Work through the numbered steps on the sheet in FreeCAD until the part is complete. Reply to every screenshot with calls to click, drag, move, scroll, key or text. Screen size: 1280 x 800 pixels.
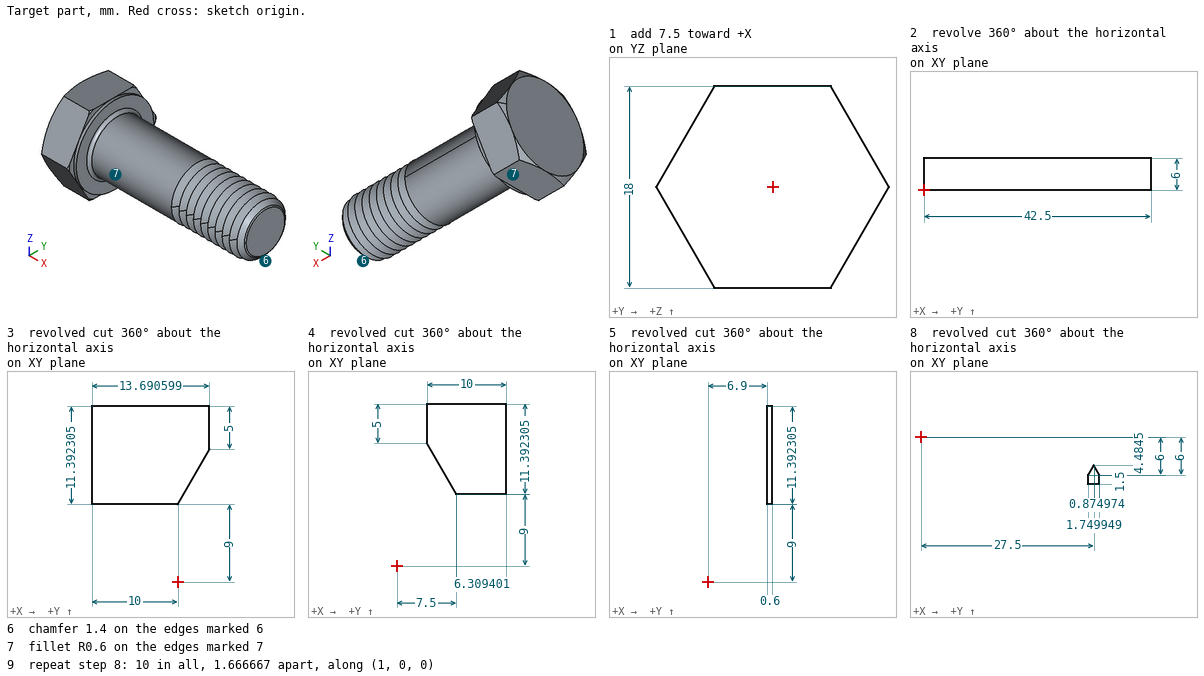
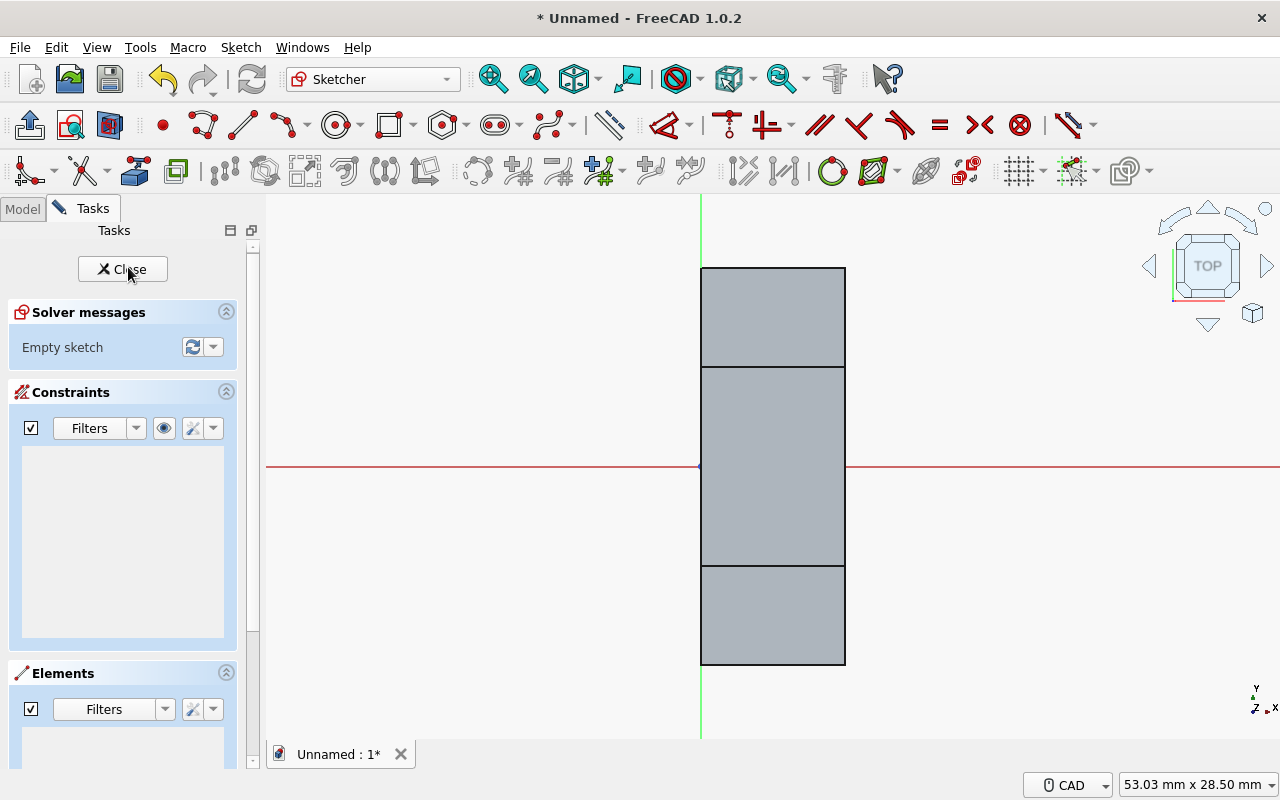
key(q)
key(s)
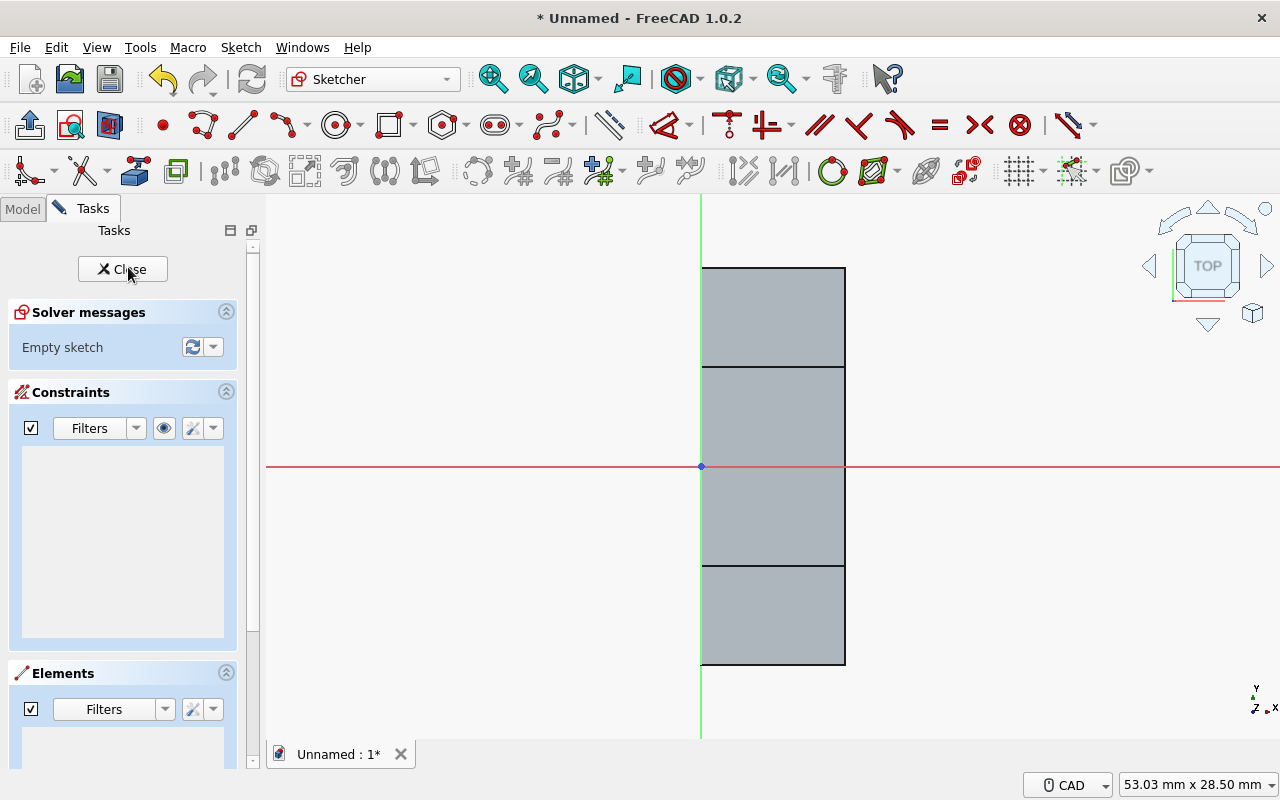
scroll(294, 536, down, 3)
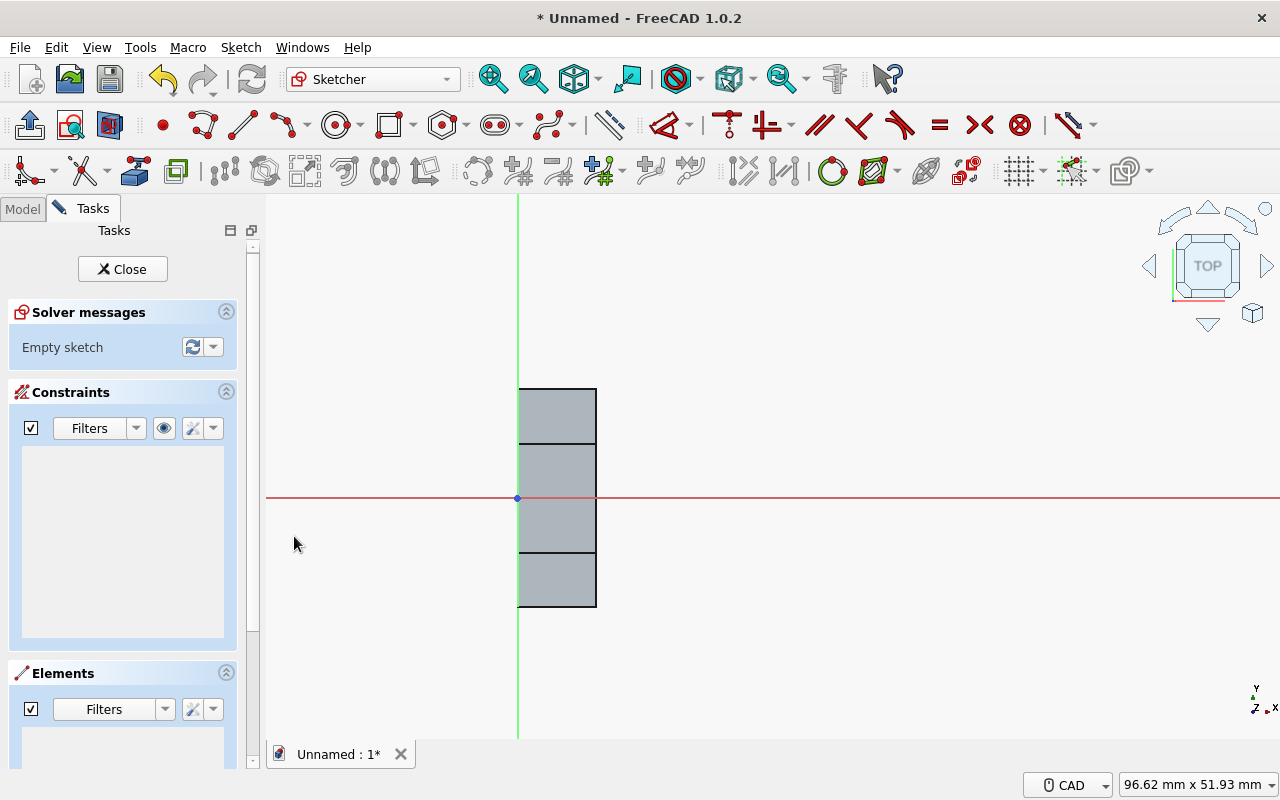
key(g)
key(r)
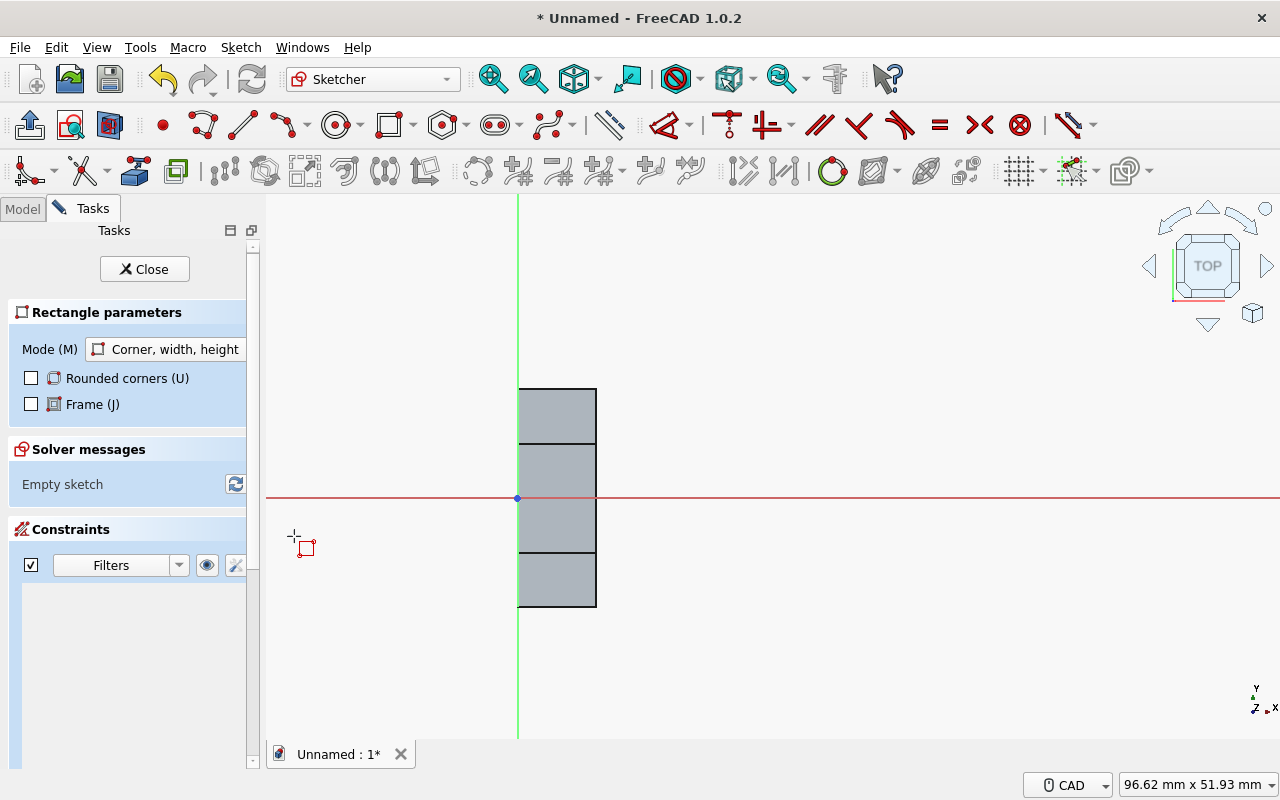
click(518, 498)
click(964, 435)
key(Escape)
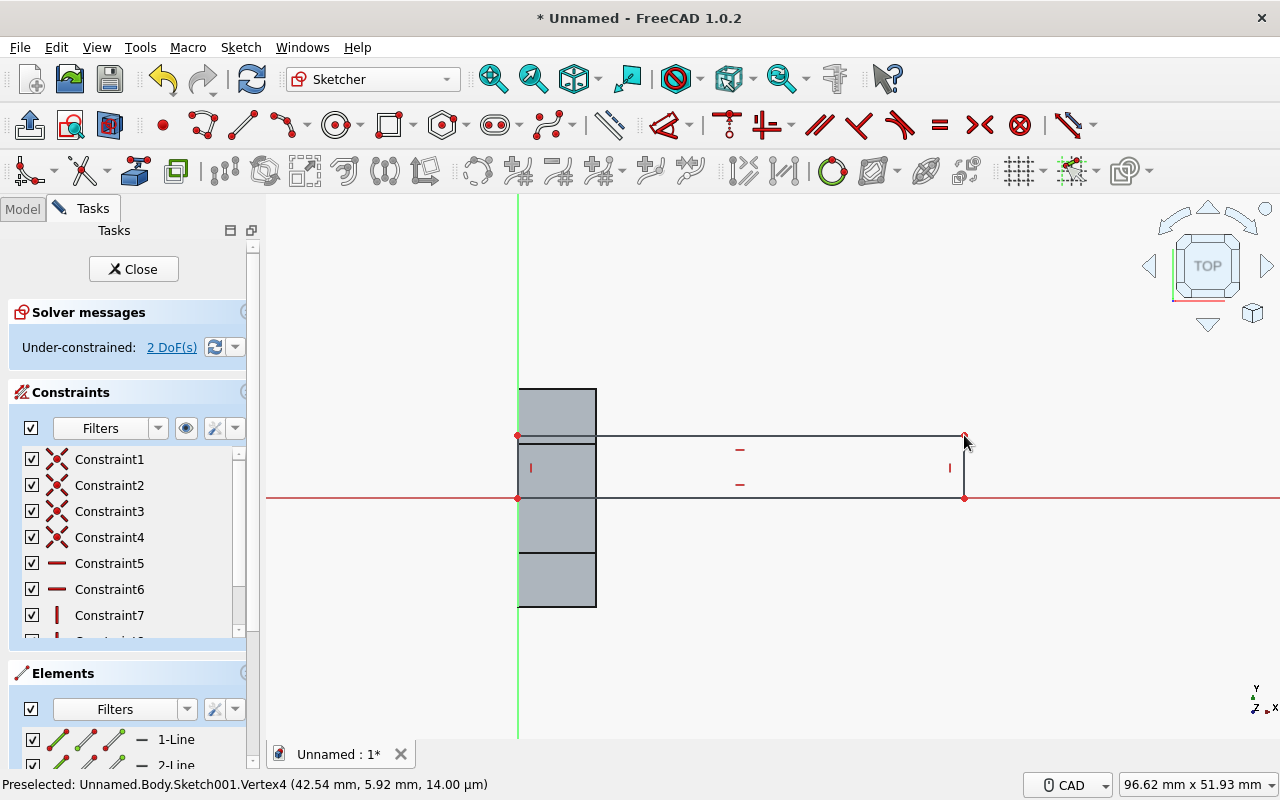
click(964, 479)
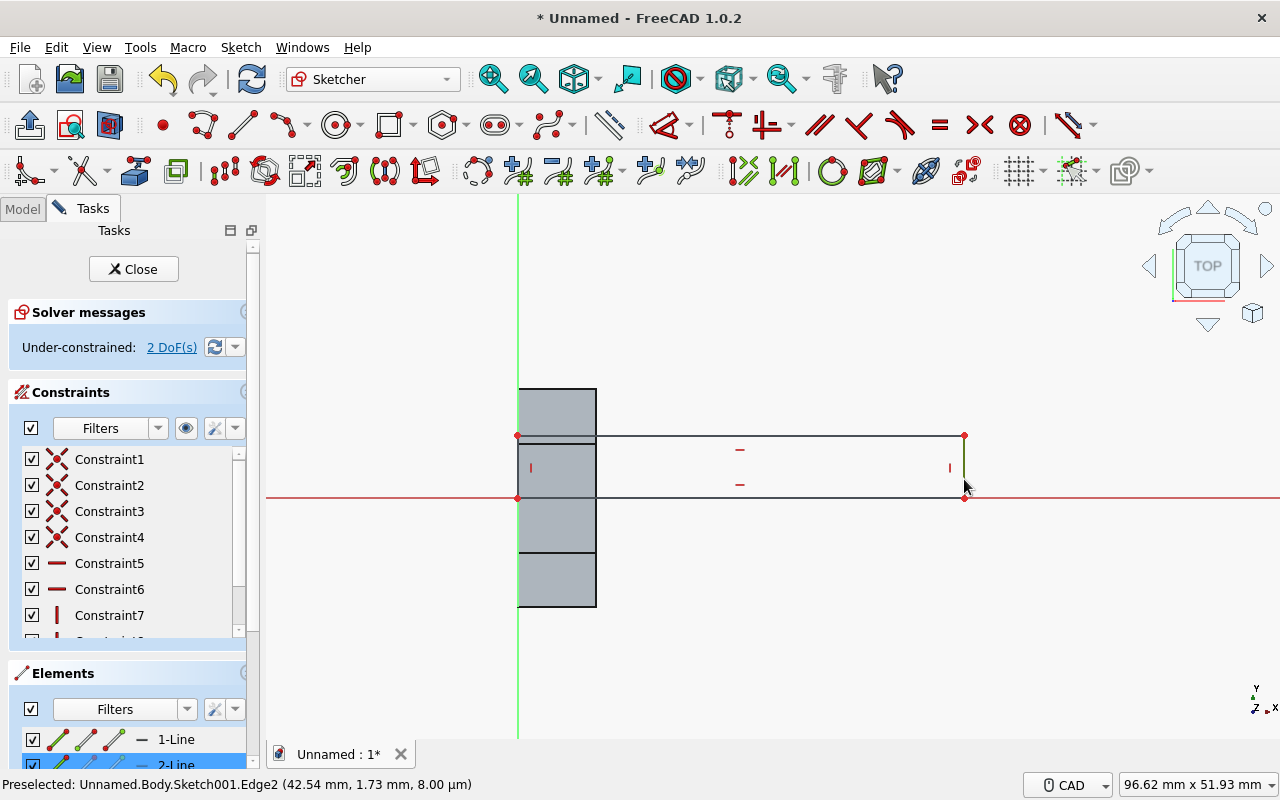
key(i)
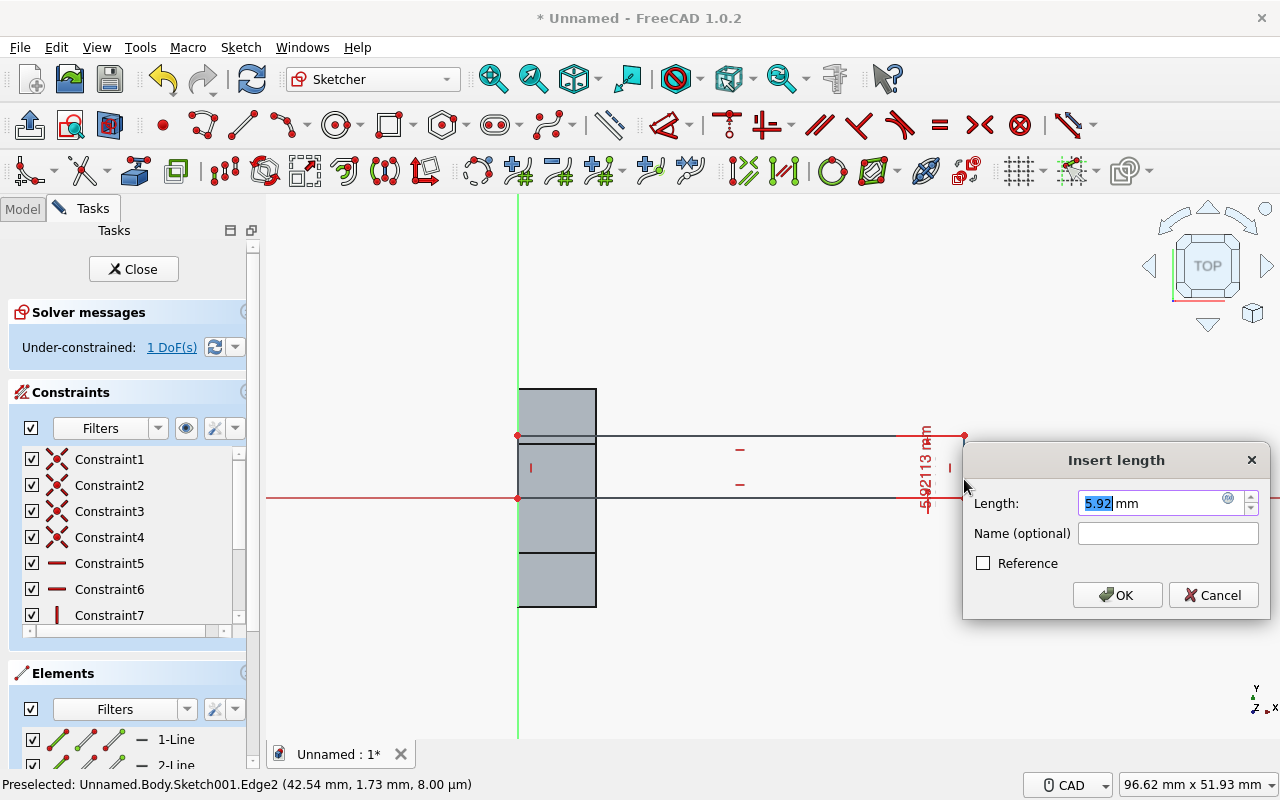
text(6)
key(Return)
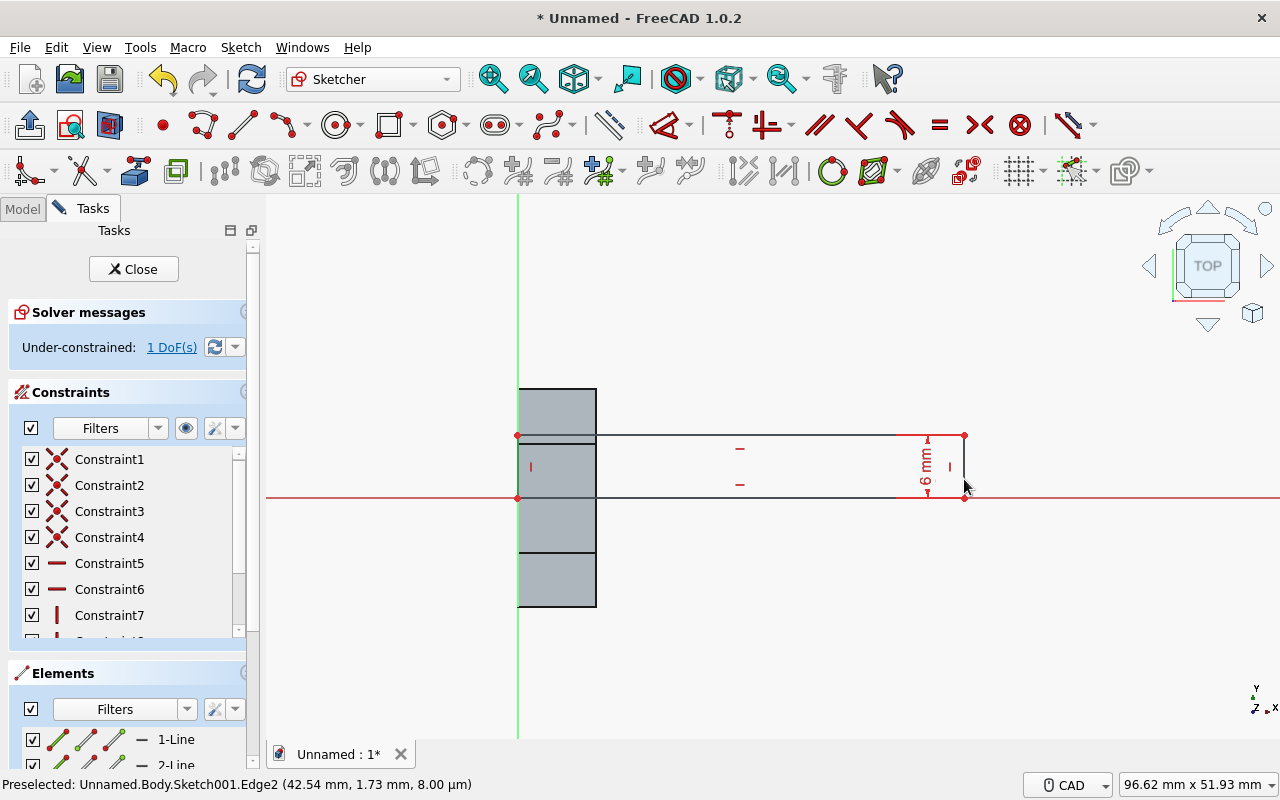
click(651, 498)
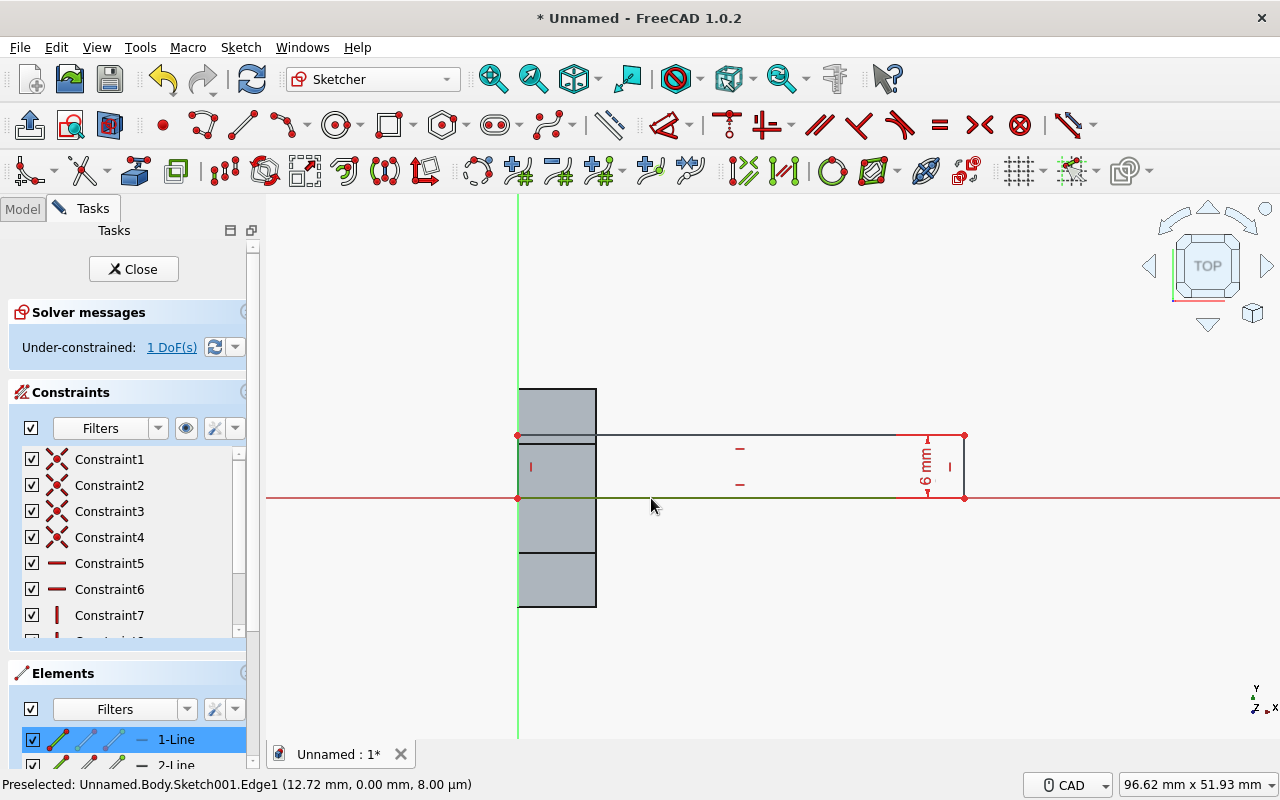
key(l)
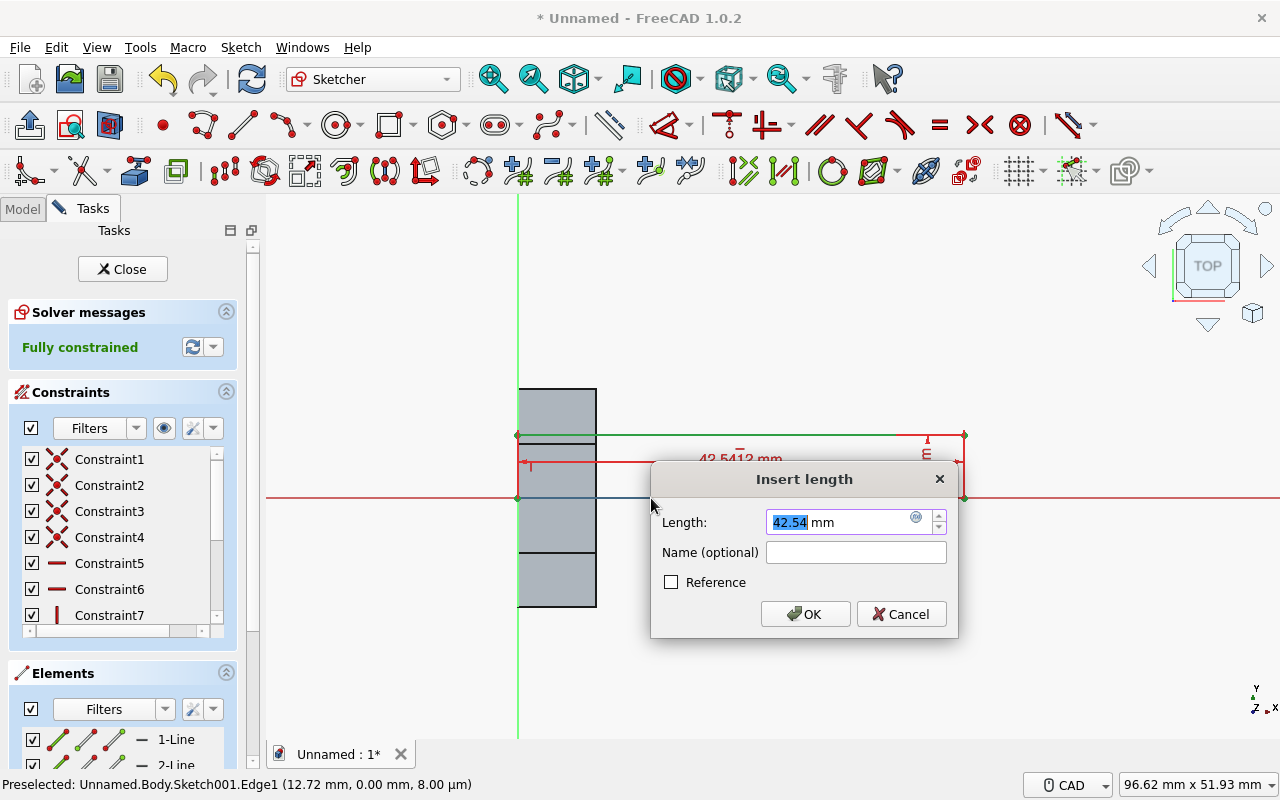
text(42.5)
key(Return)